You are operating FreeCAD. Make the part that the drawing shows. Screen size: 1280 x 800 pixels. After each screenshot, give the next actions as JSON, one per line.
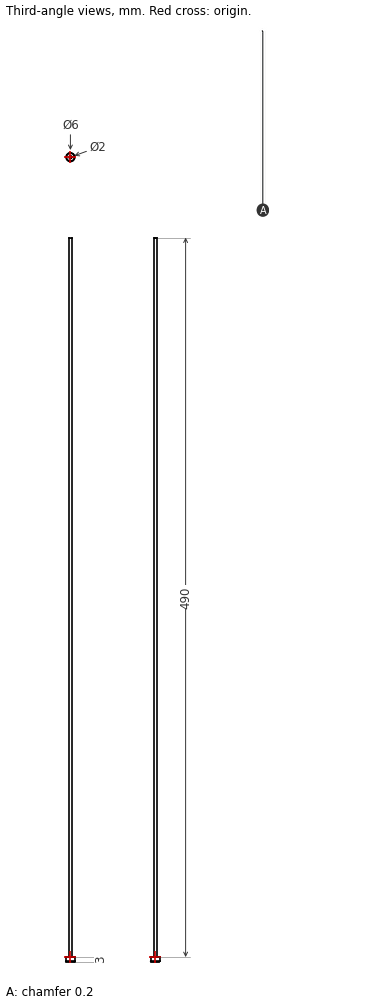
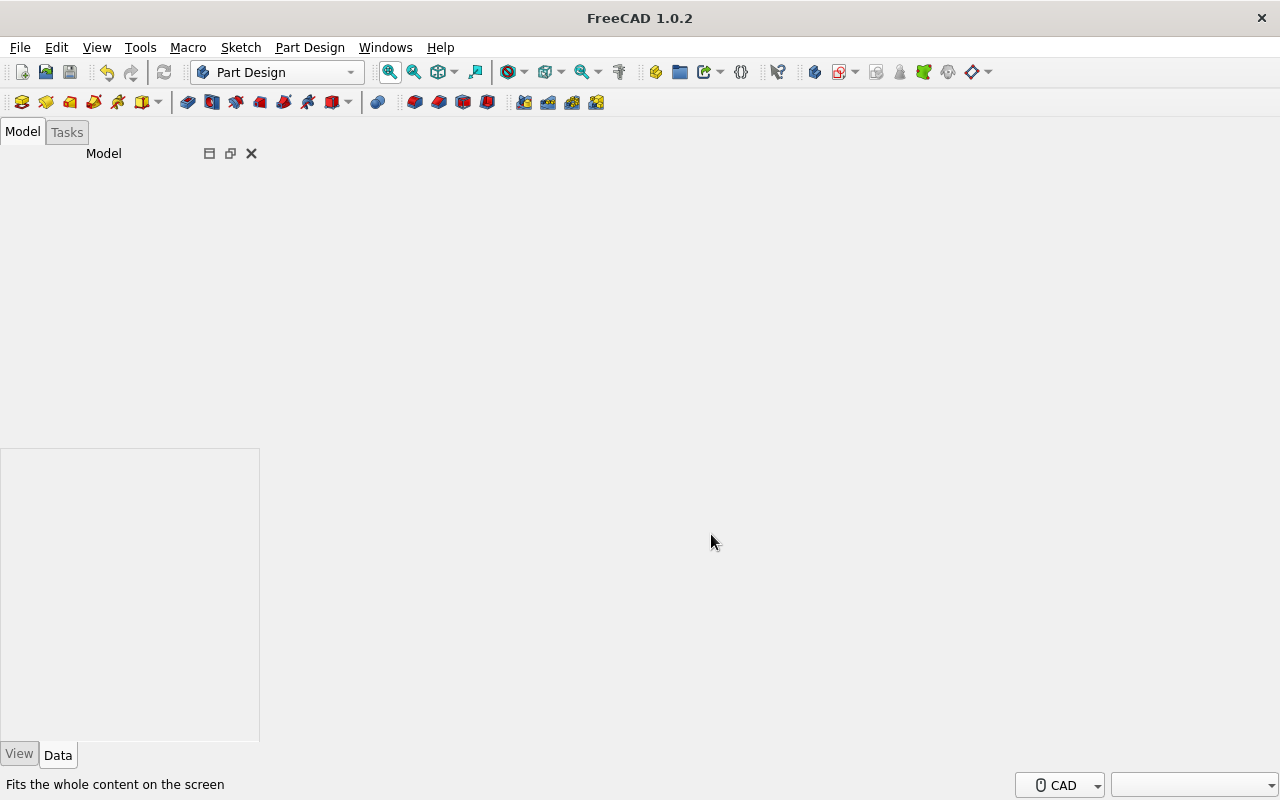
{"action": "key", "text": "ctrl+n"}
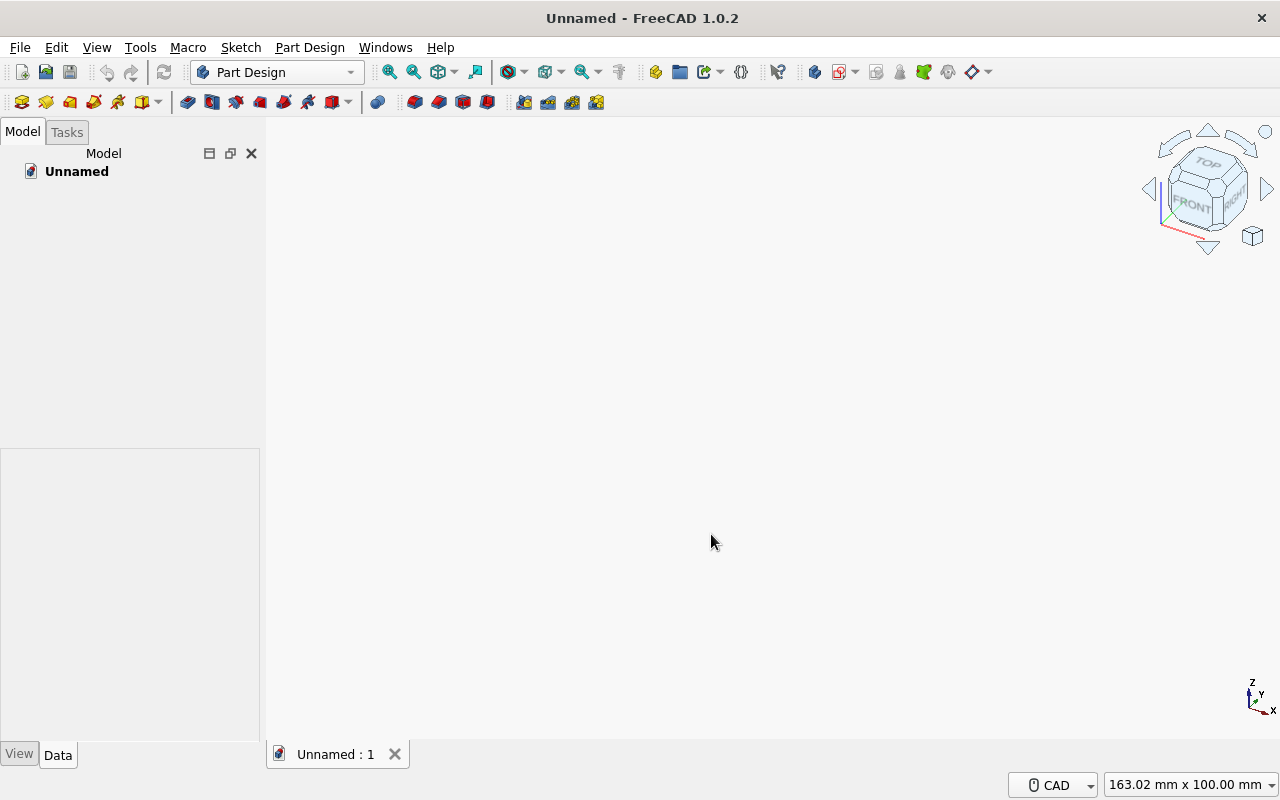
{"action": "left_click", "coordinate": [840, 72]}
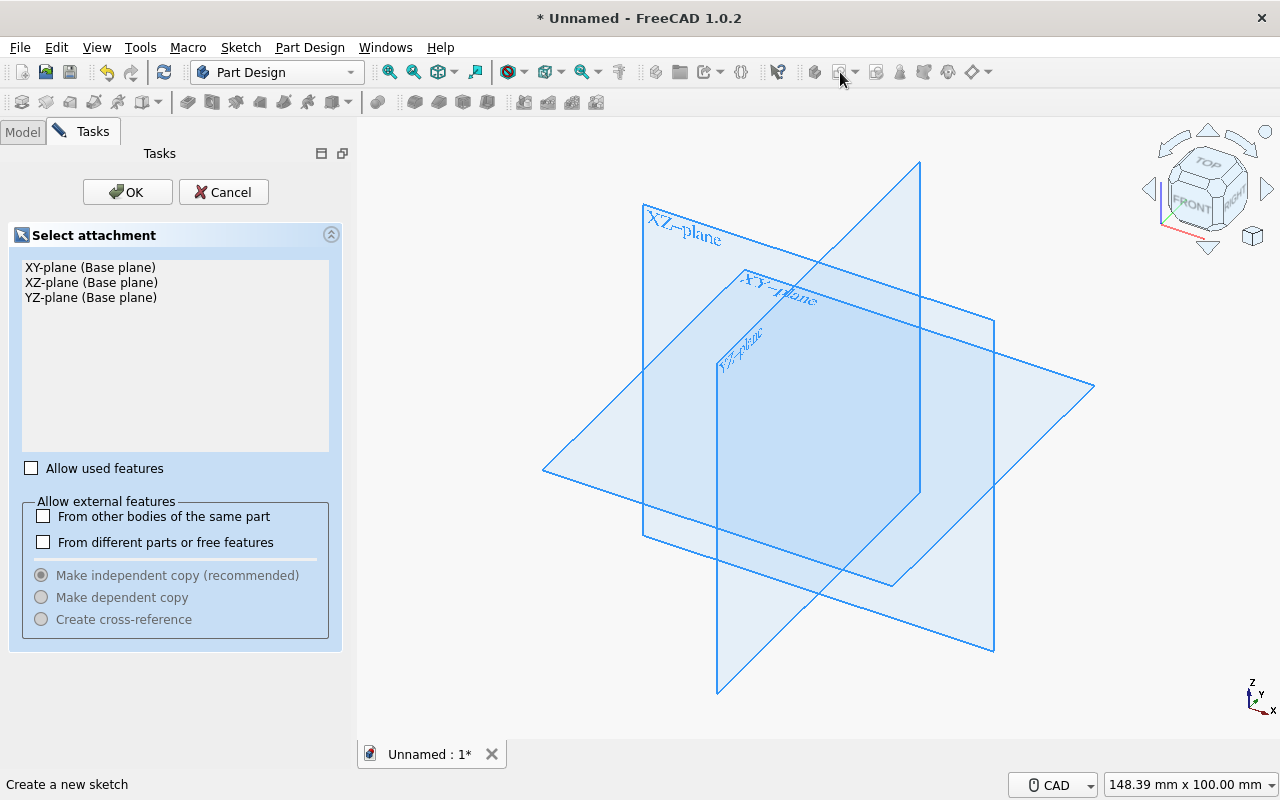
{"action": "left_click", "coordinate": [82, 268]}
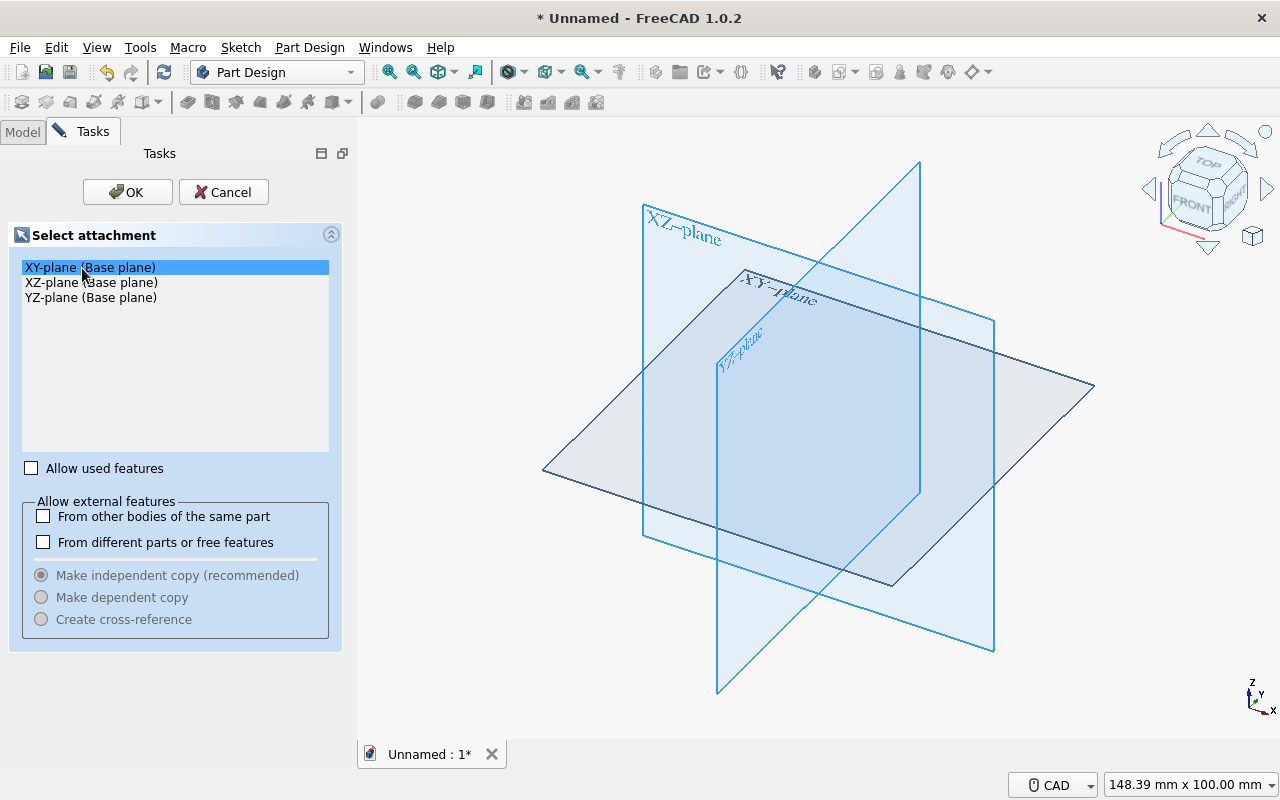
{"action": "left_click", "coordinate": [128, 192]}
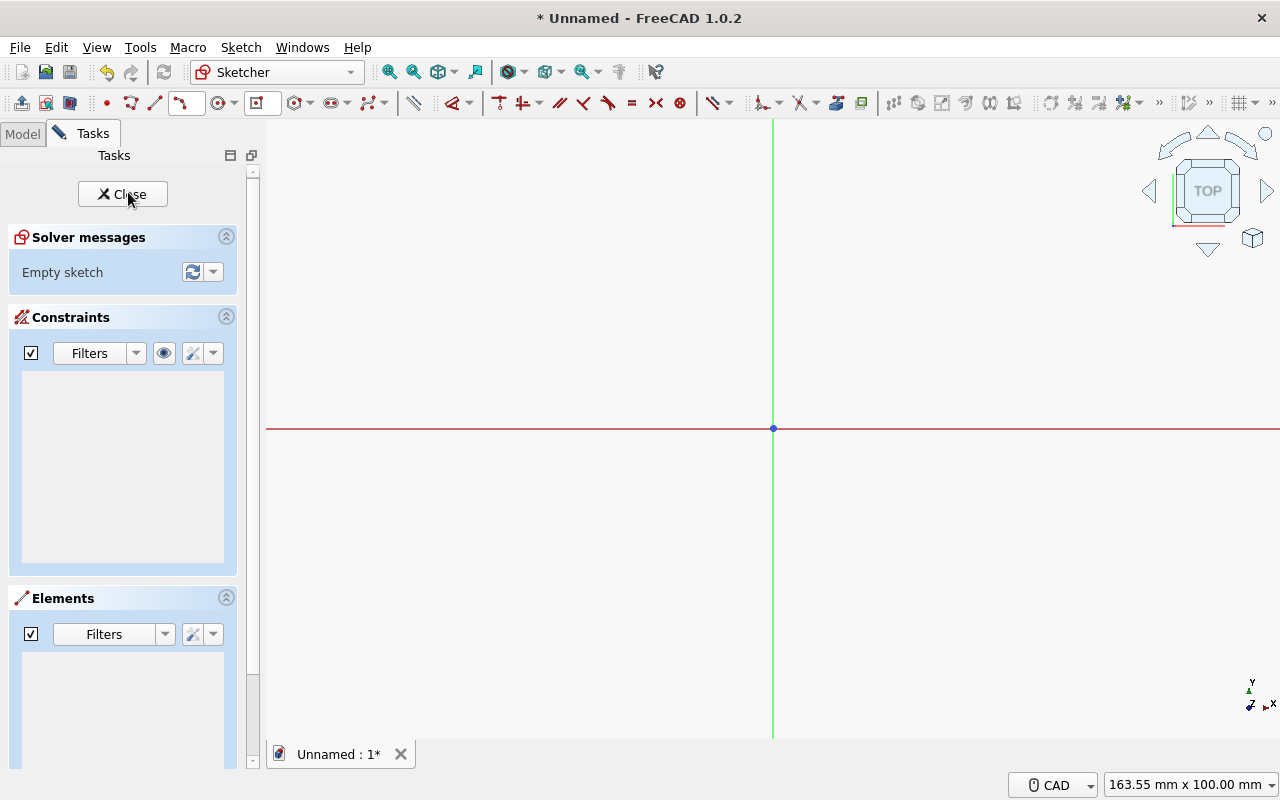
{"action": "scroll", "coordinate": [777, 429], "scroll_direction": "up", "scroll_amount": 15}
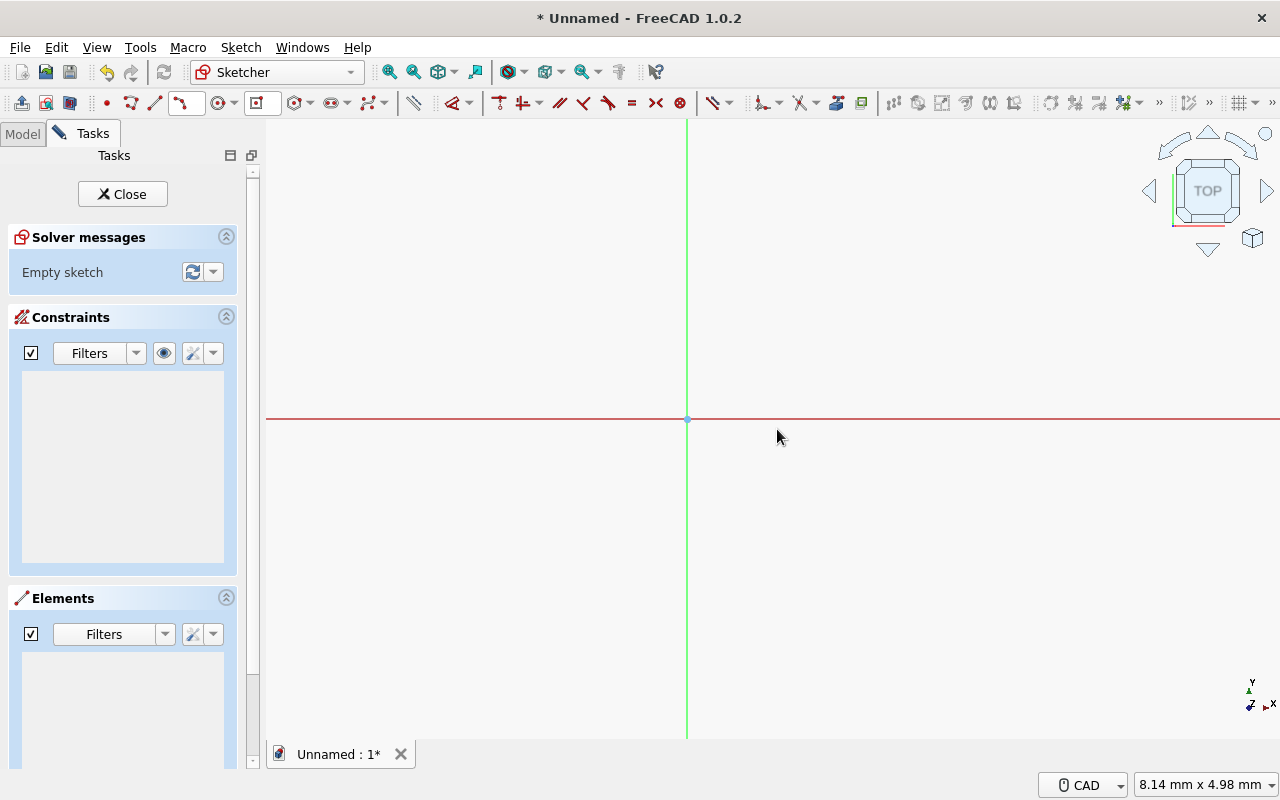
{"action": "scroll", "coordinate": [652, 400], "scroll_direction": "up", "scroll_amount": 2}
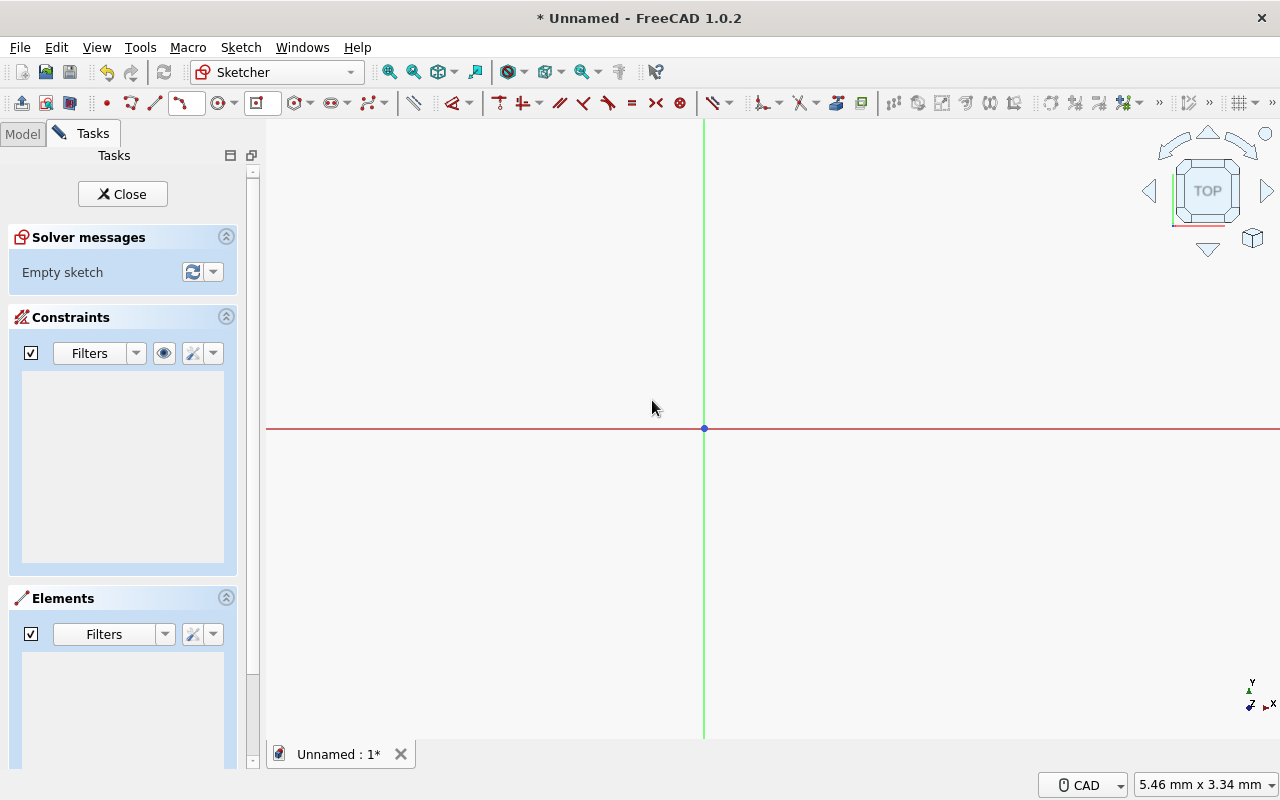
{"action": "key", "text": "g c"}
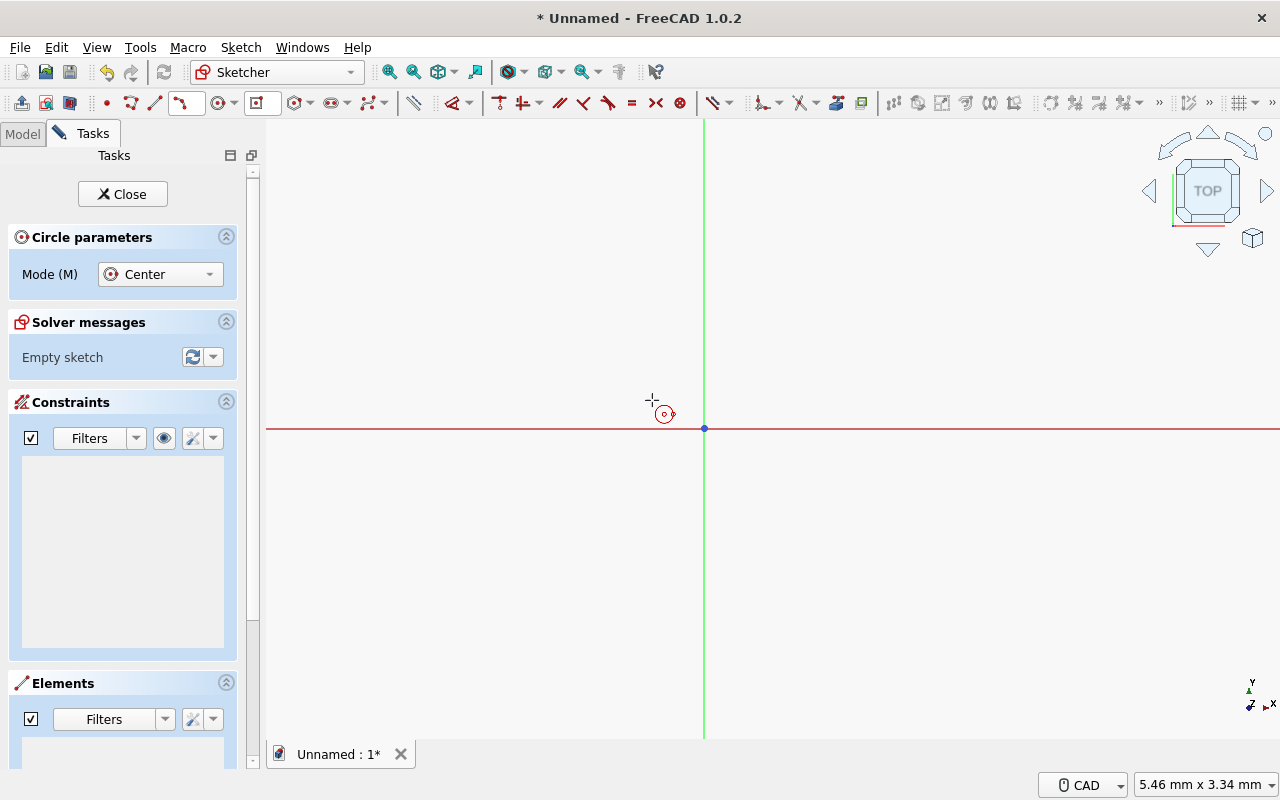
{"action": "left_click", "coordinate": [704, 429]}
{"action": "left_click", "coordinate": [835, 297]}
{"action": "key", "text": "Escape"}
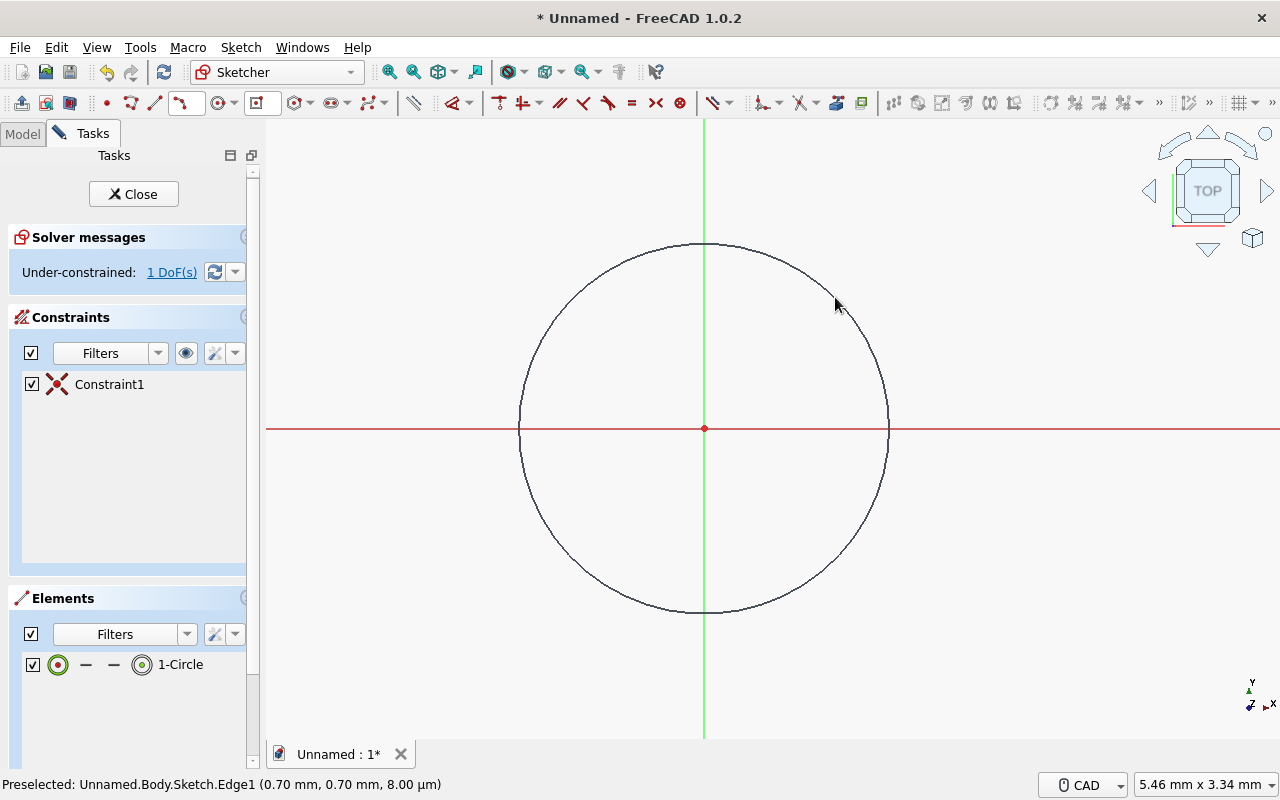
{"action": "key", "text": "d"}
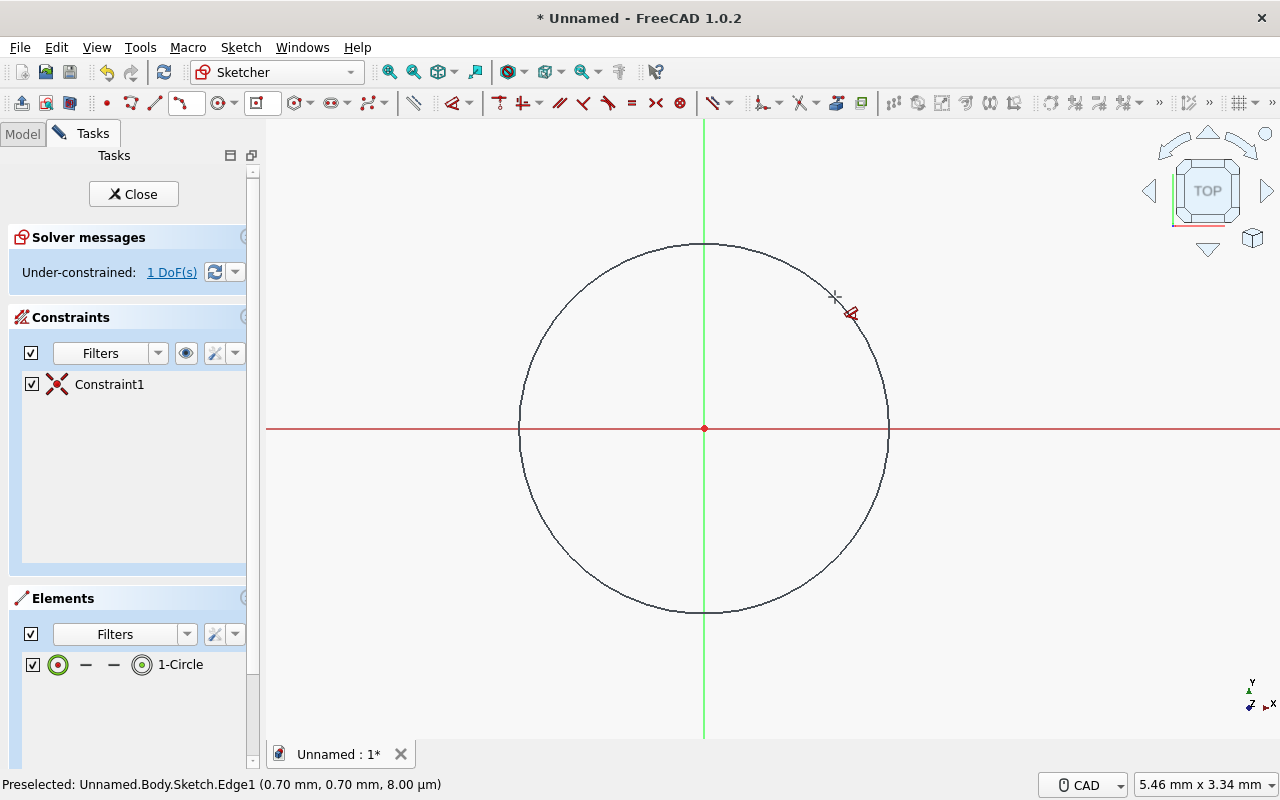
{"action": "left_click", "coordinate": [835, 298]}
{"action": "left_click", "coordinate": [858, 275]}